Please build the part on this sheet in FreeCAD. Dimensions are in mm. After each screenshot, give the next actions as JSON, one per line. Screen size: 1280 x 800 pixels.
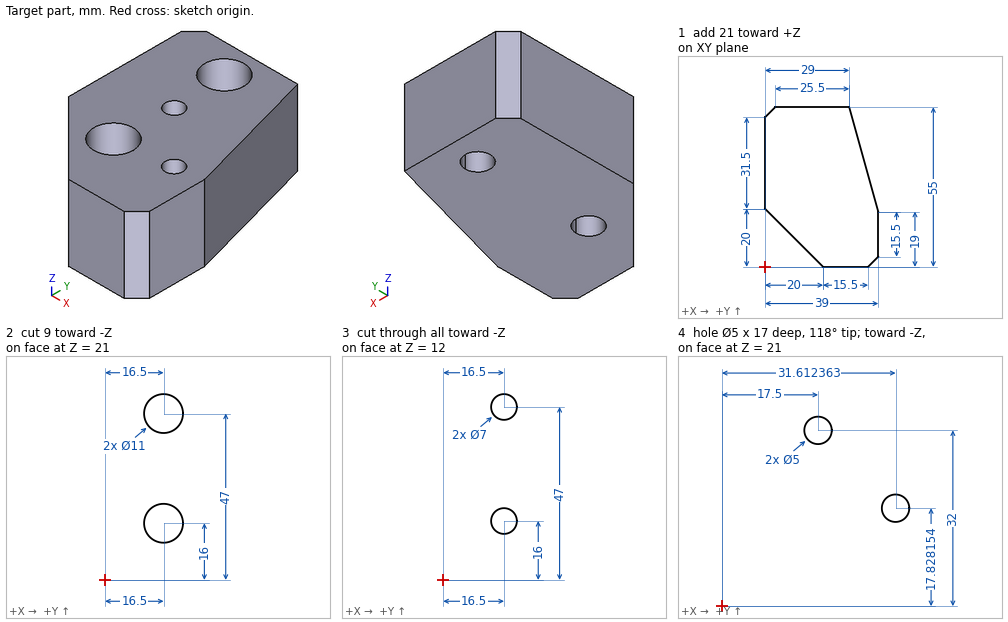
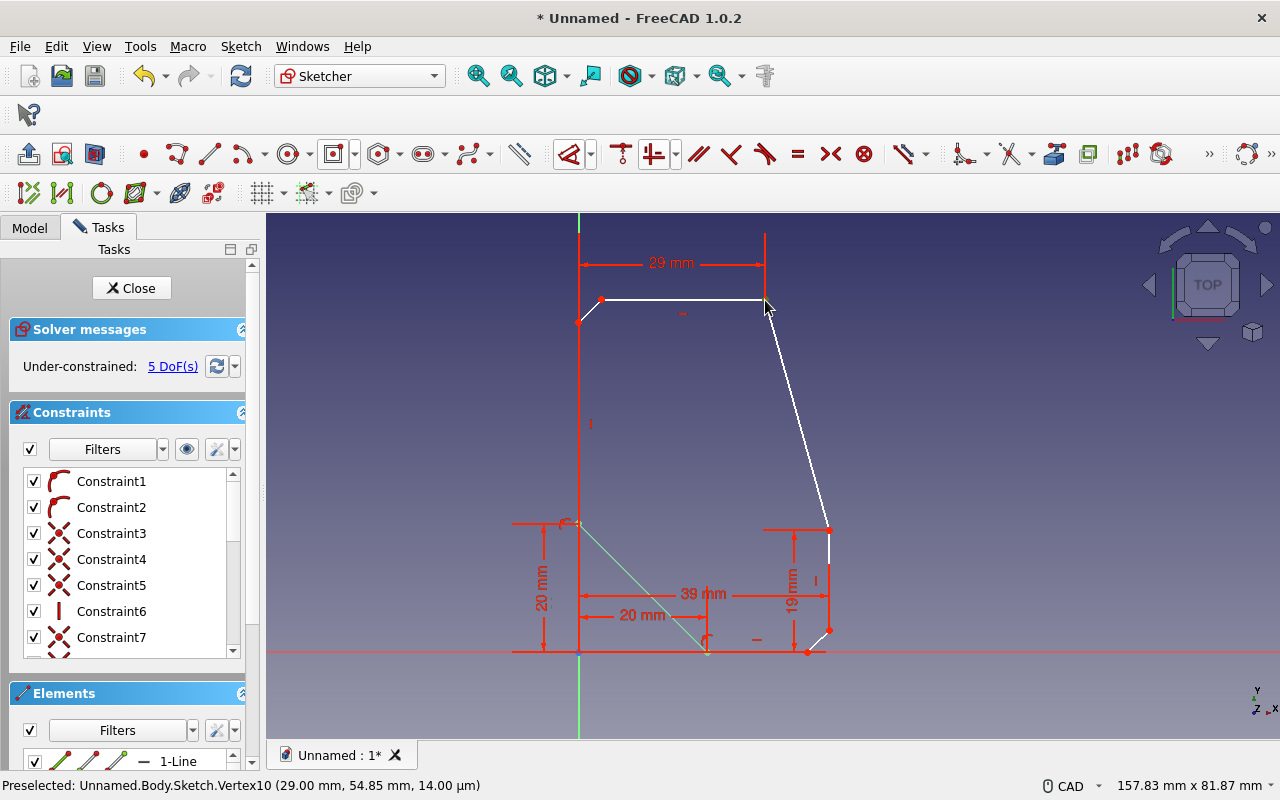
{"action": "key", "text": "i"}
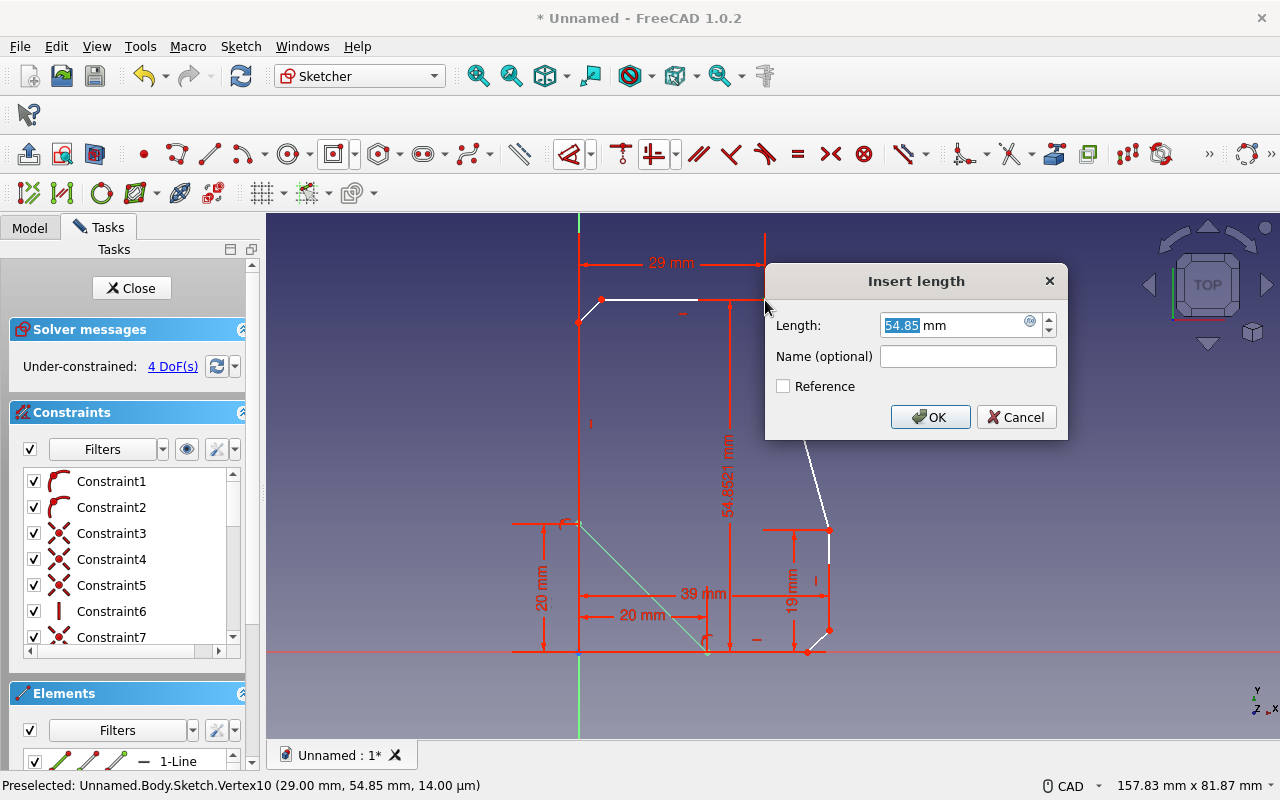
{"action": "type", "text": "55"}
{"action": "key", "text": "Return"}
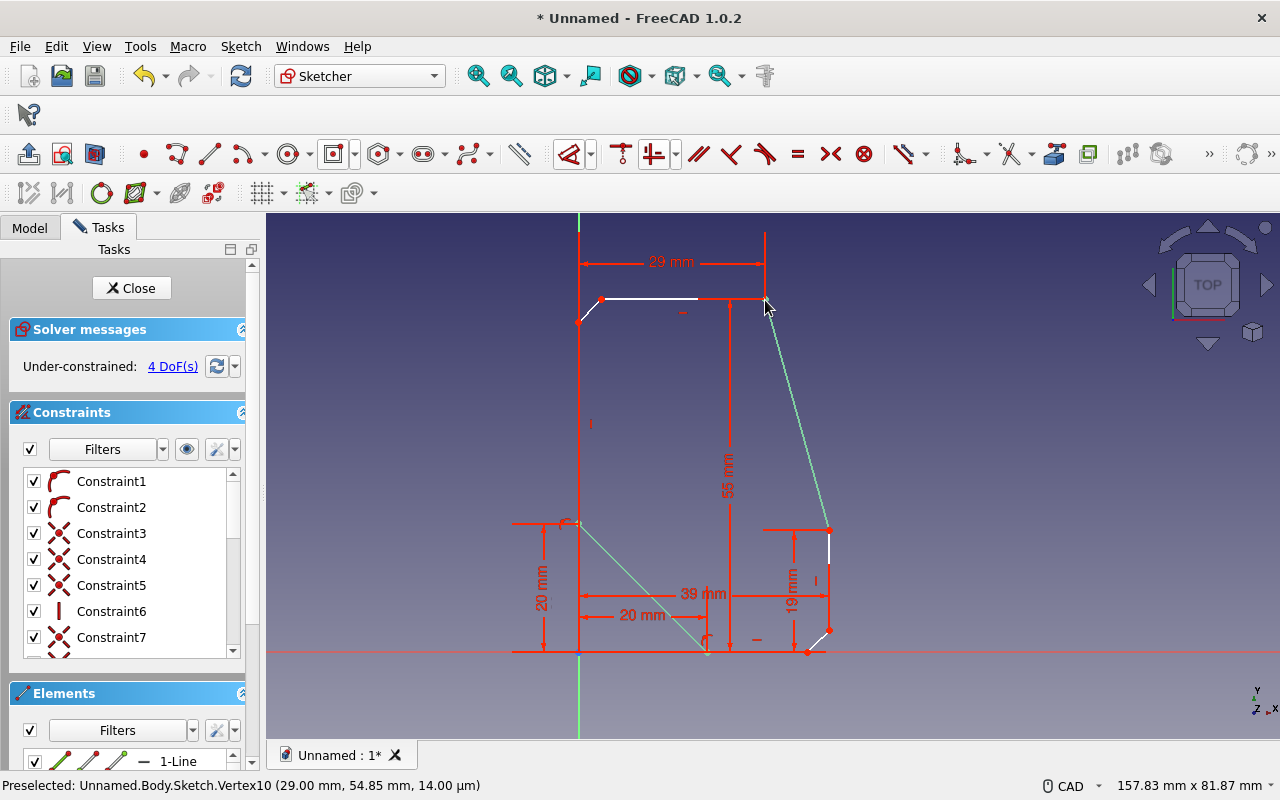
{"action": "left_click", "coordinate": [737, 652]}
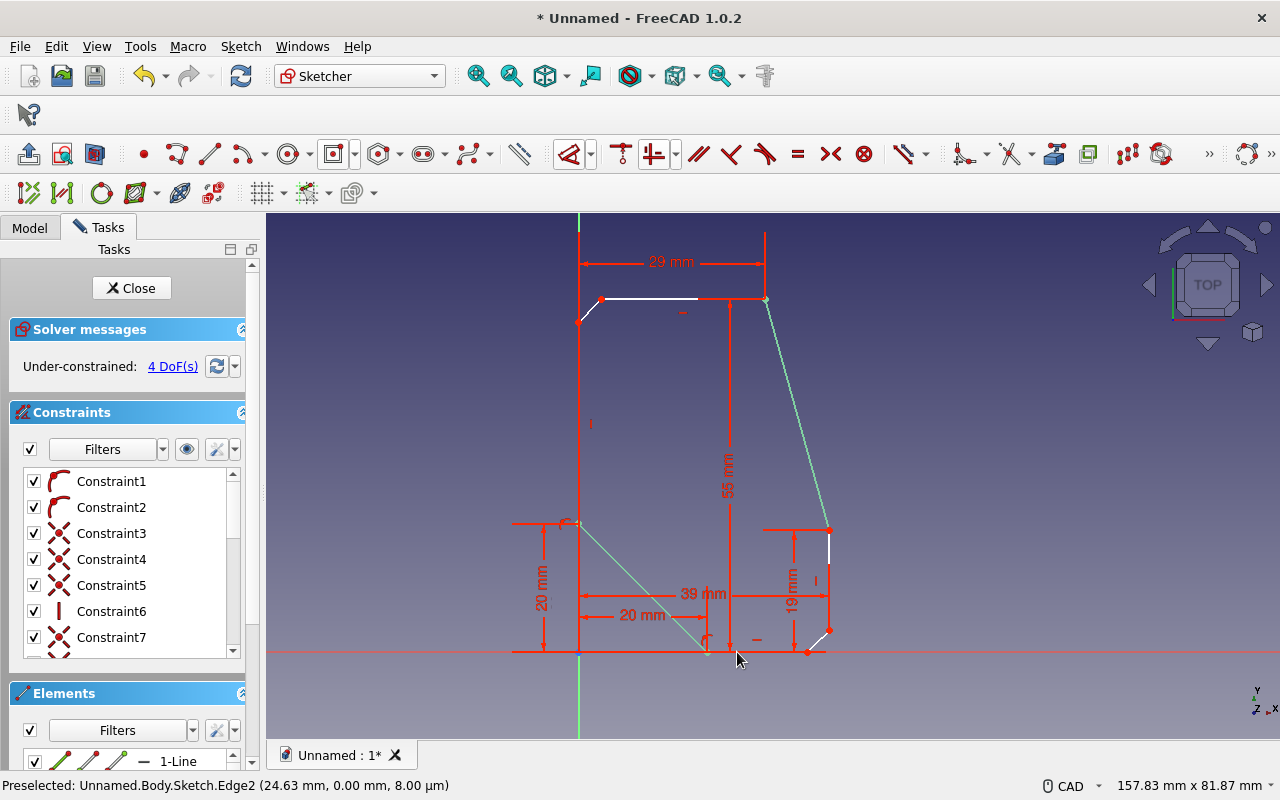
{"action": "key", "text": "l"}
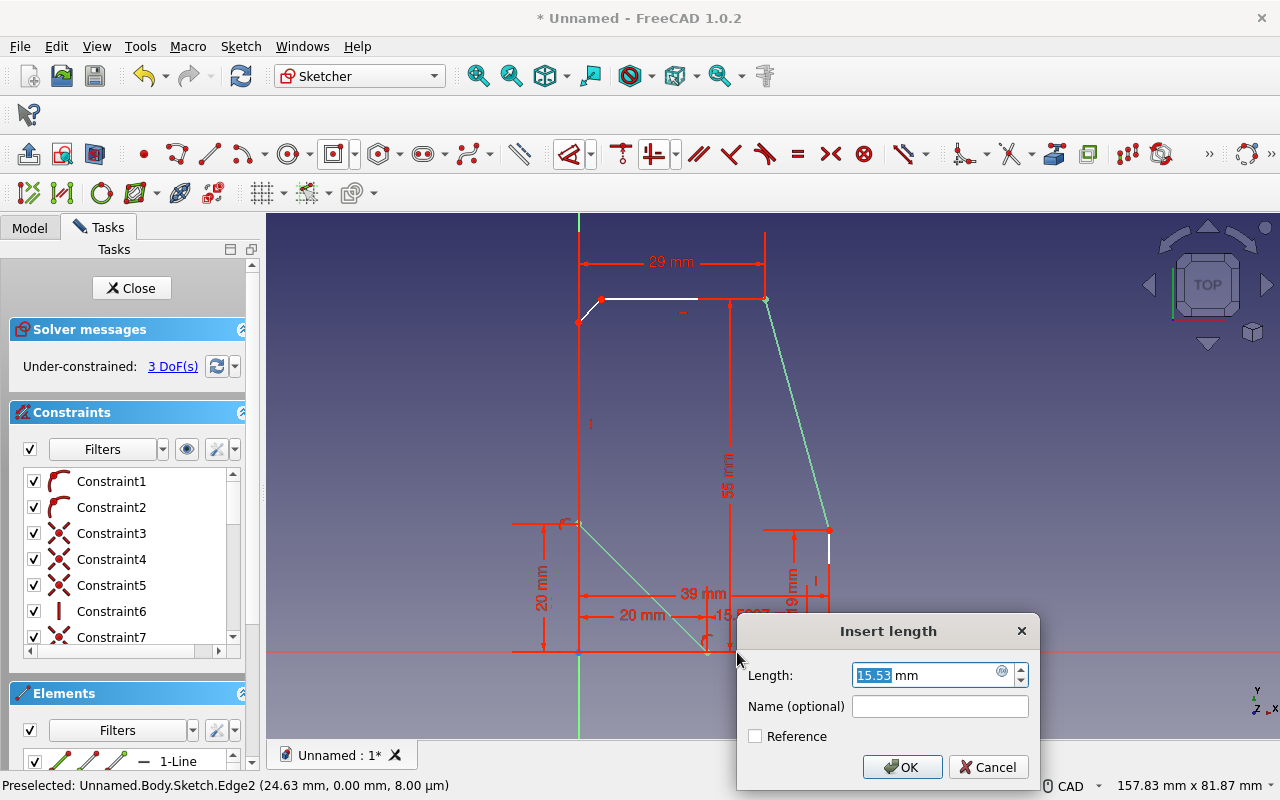
{"action": "type", "text": "15.5"}
{"action": "key", "text": "Return"}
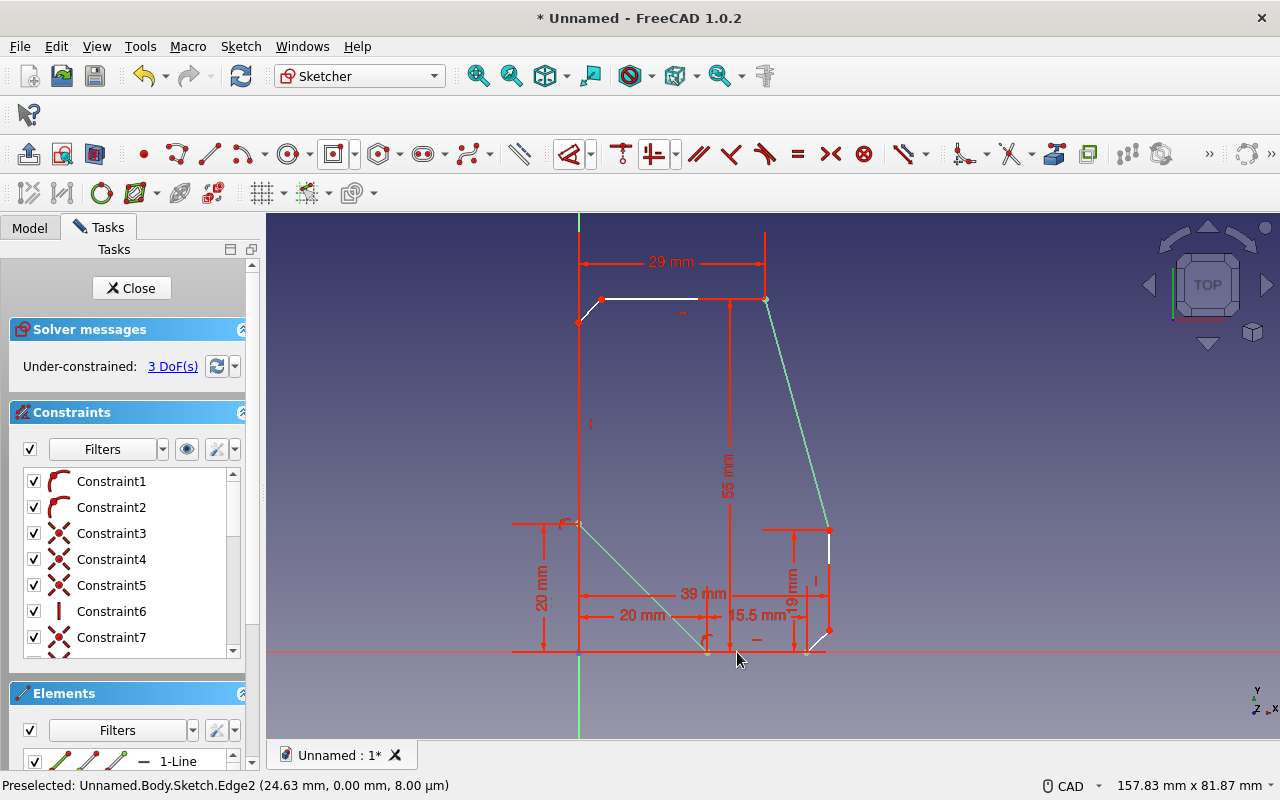
{"action": "left_click", "coordinate": [829, 601]}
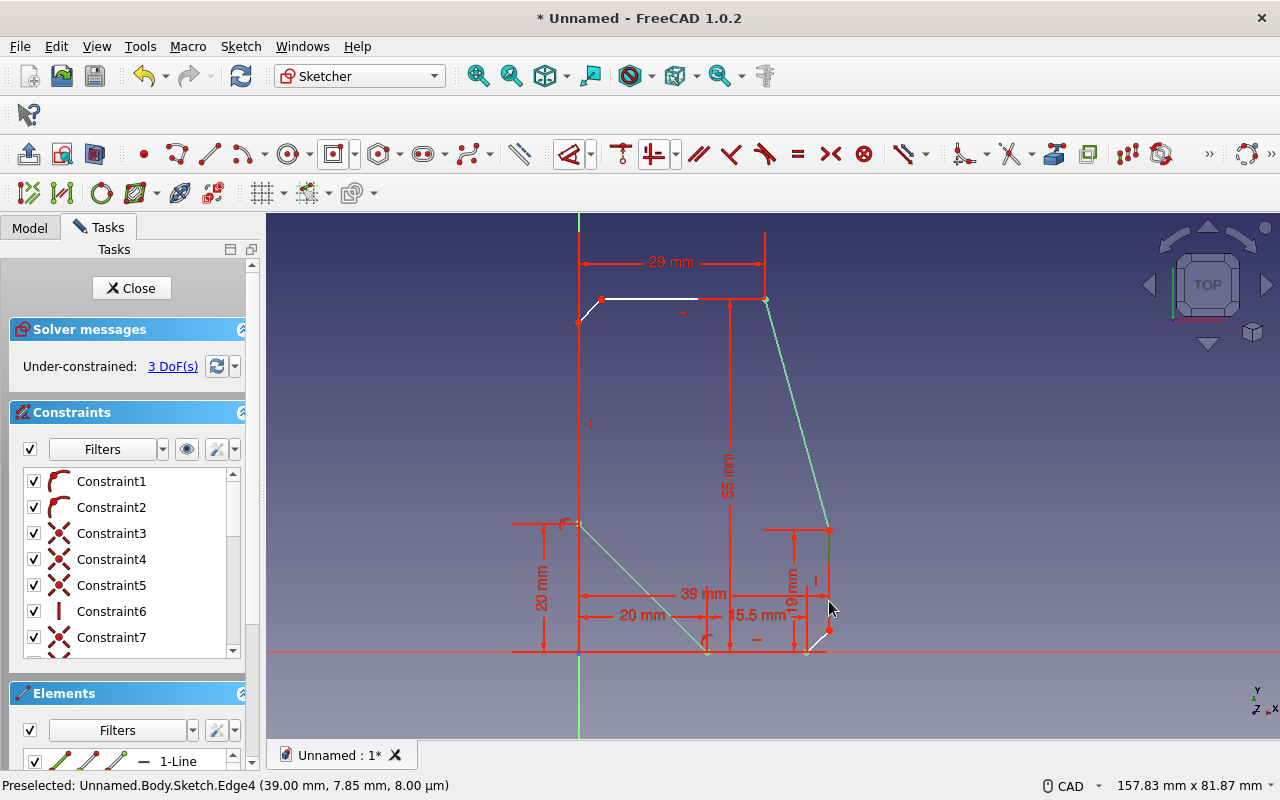
{"action": "key", "text": "i"}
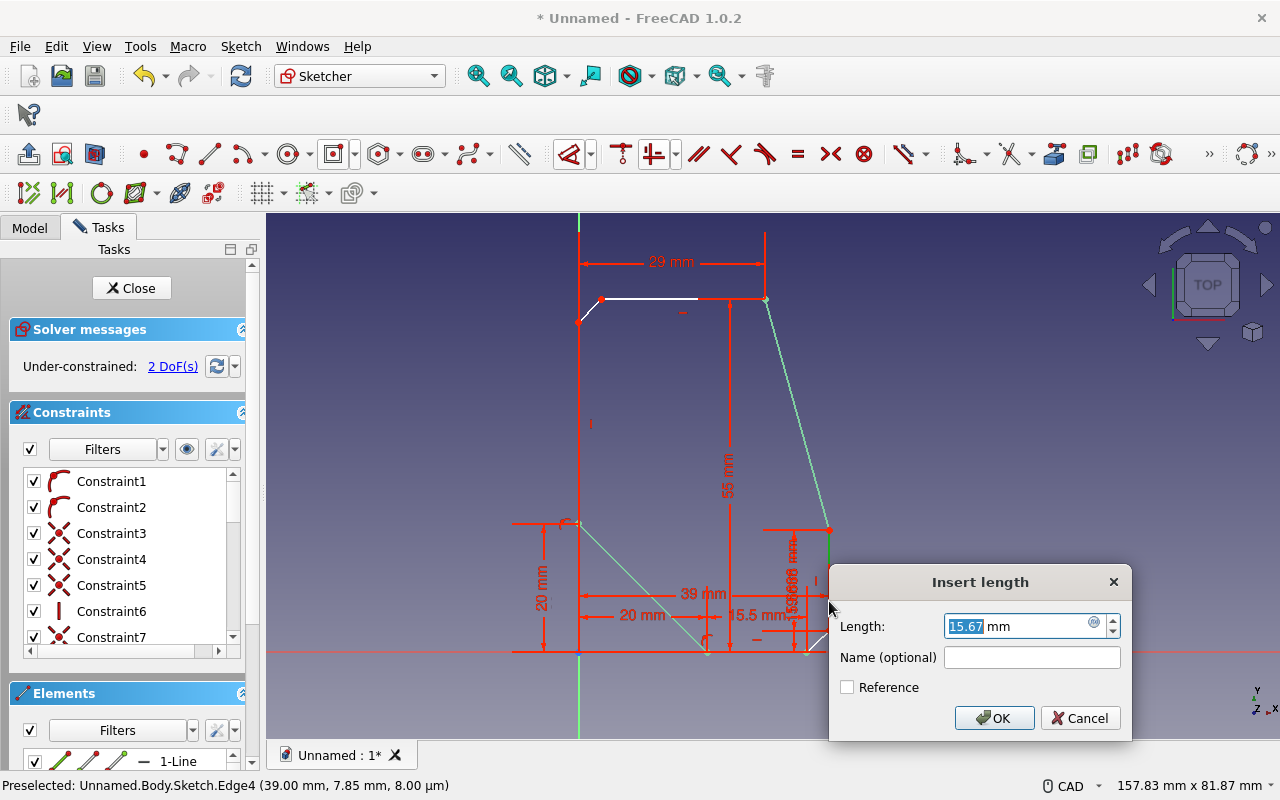
{"action": "type", "text": "15.5"}
{"action": "key", "text": "Return"}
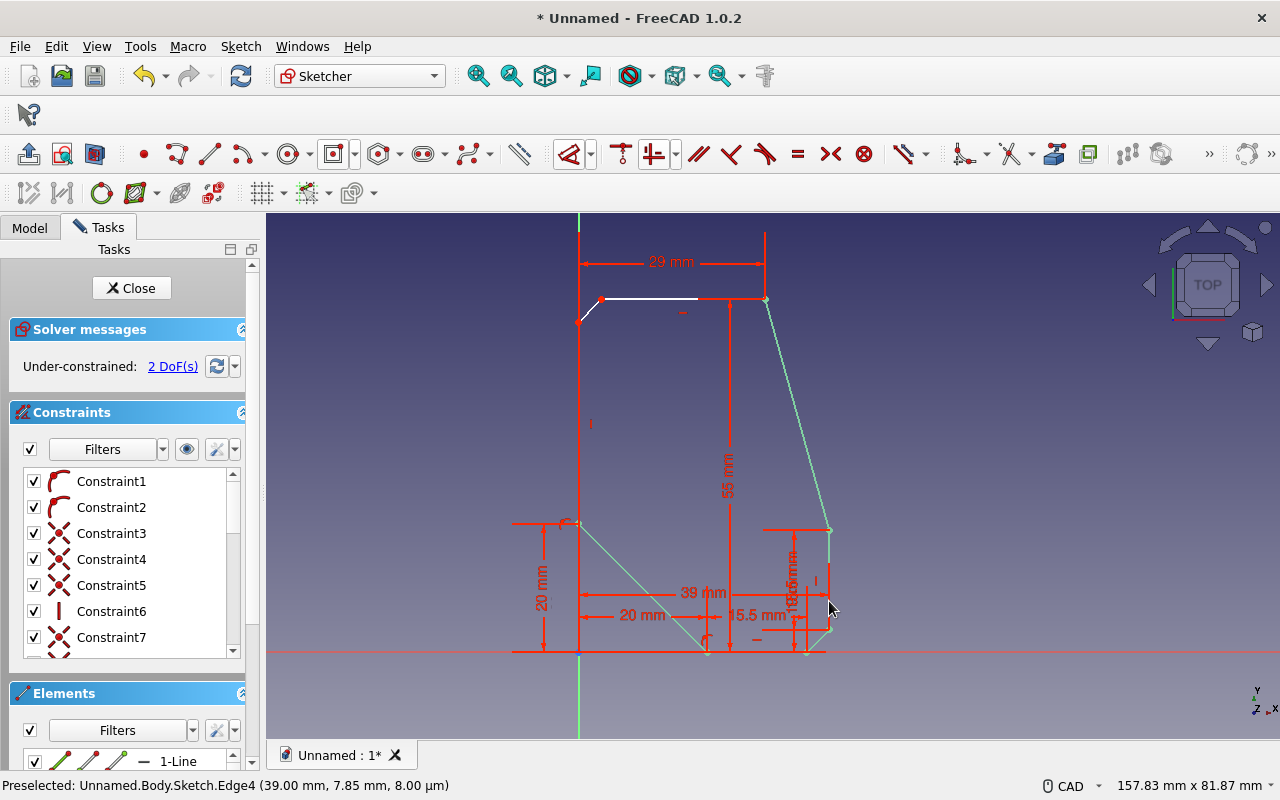
{"action": "left_click", "coordinate": [716, 299]}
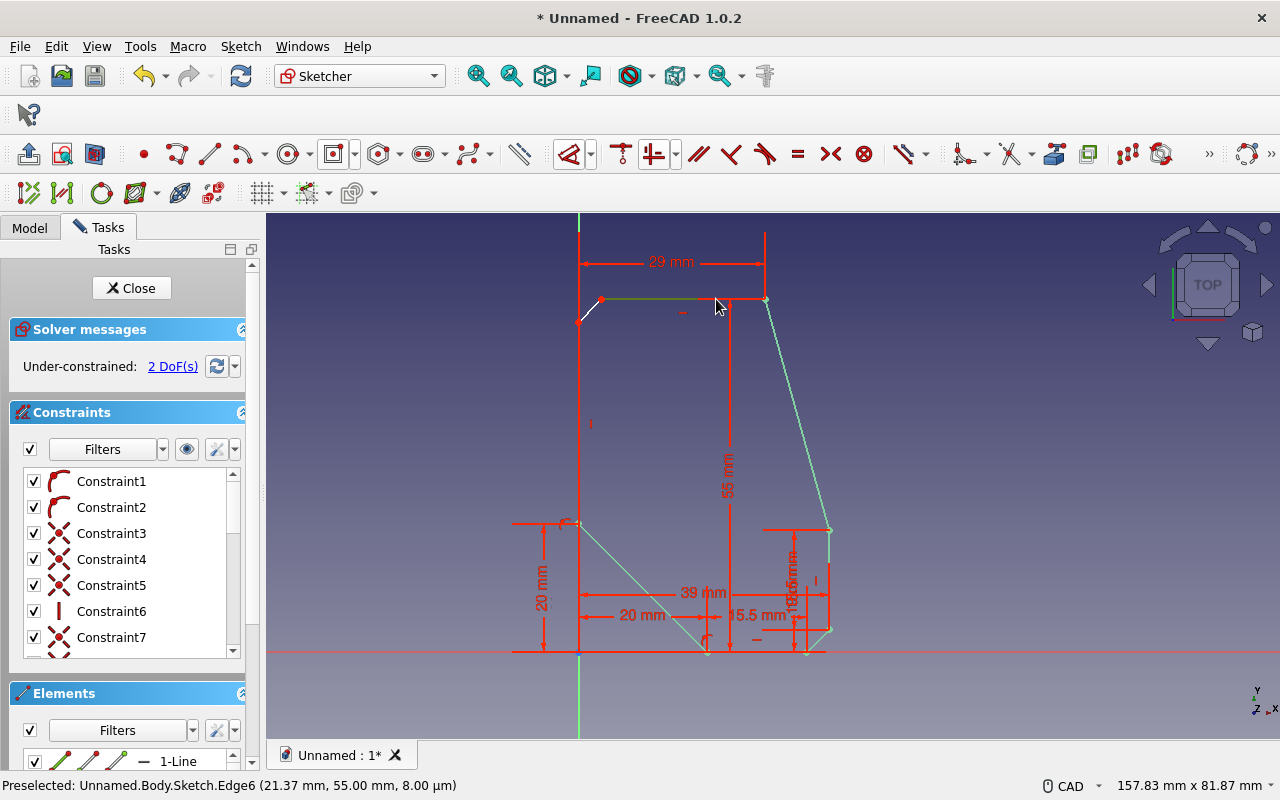
{"action": "left_click", "coordinate": [590, 154]}